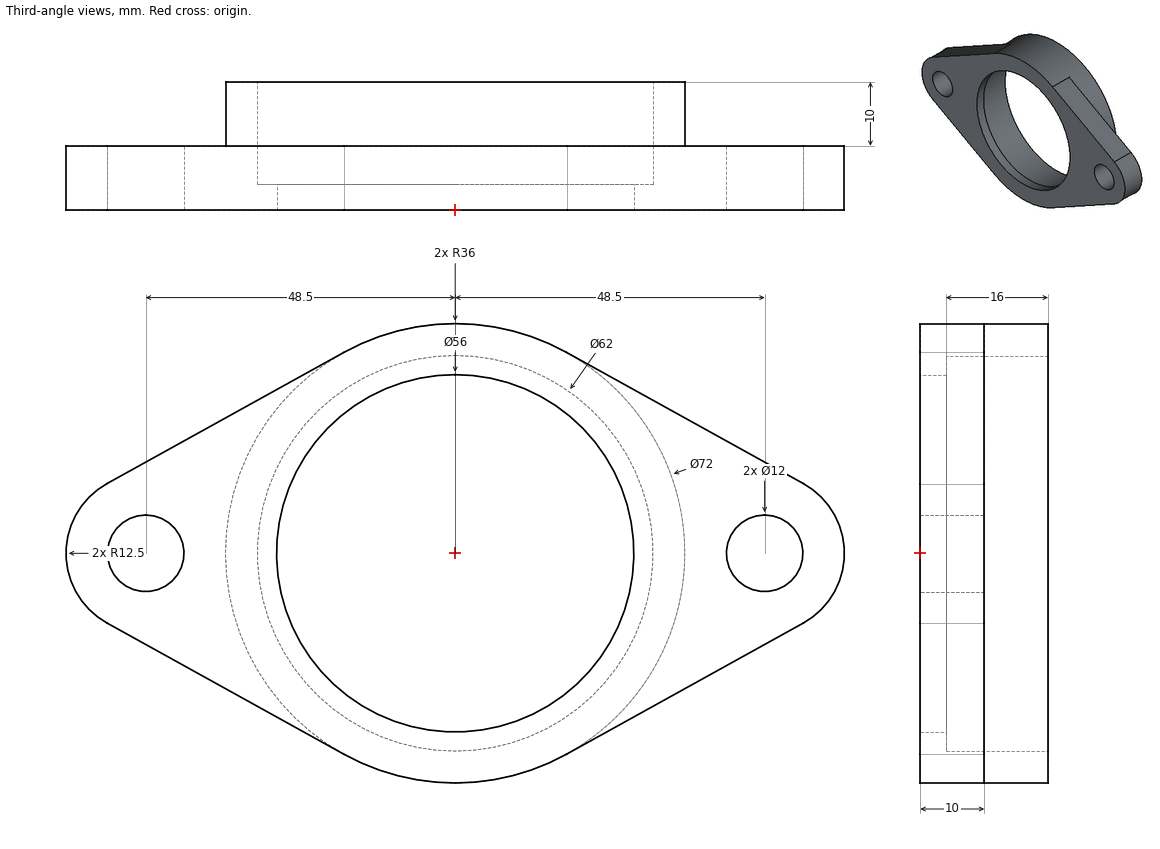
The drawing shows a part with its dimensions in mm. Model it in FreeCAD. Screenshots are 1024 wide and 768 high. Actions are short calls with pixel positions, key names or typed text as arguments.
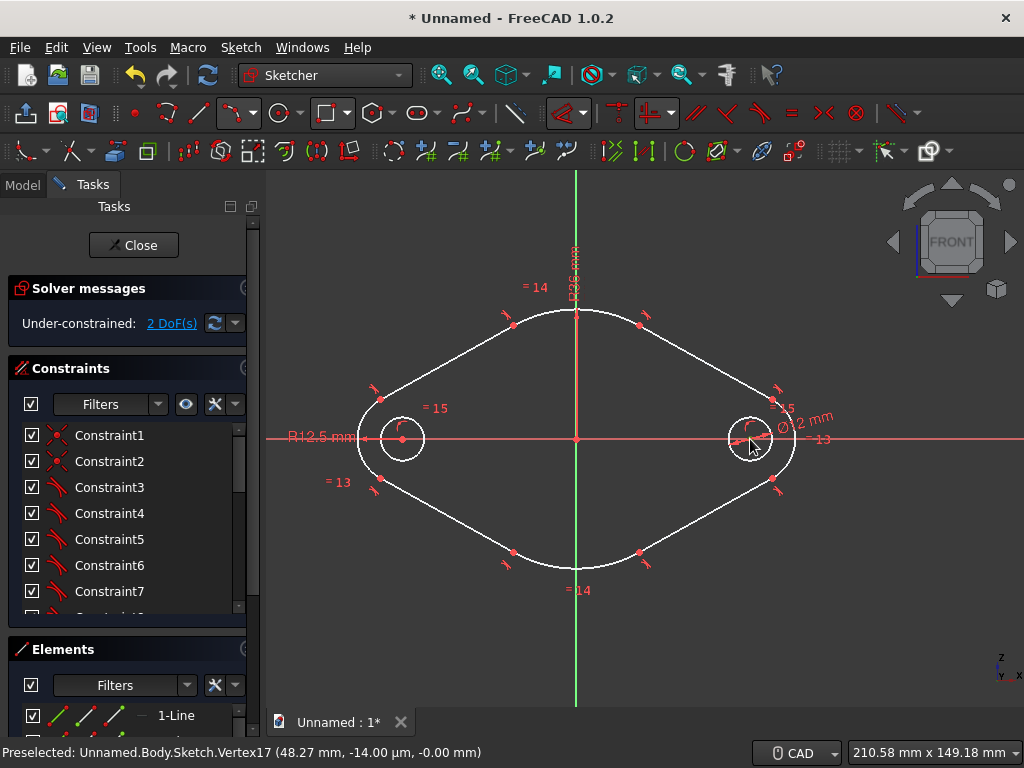
click(586, 114)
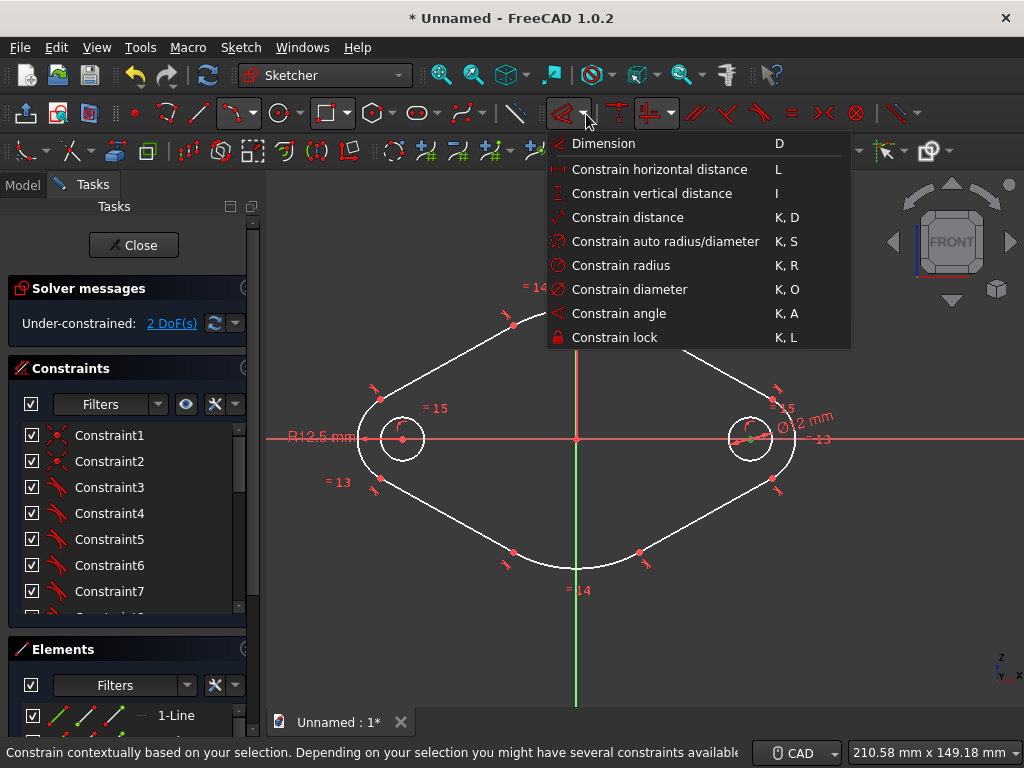
click(699, 169)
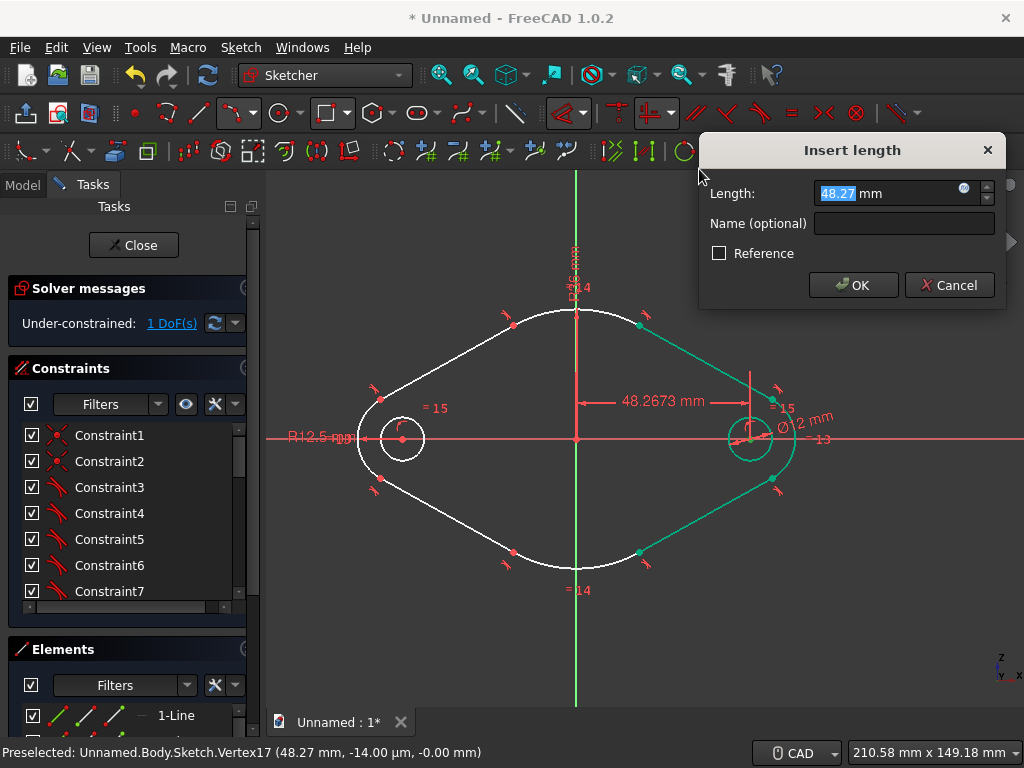
text(48.5)
key(Return)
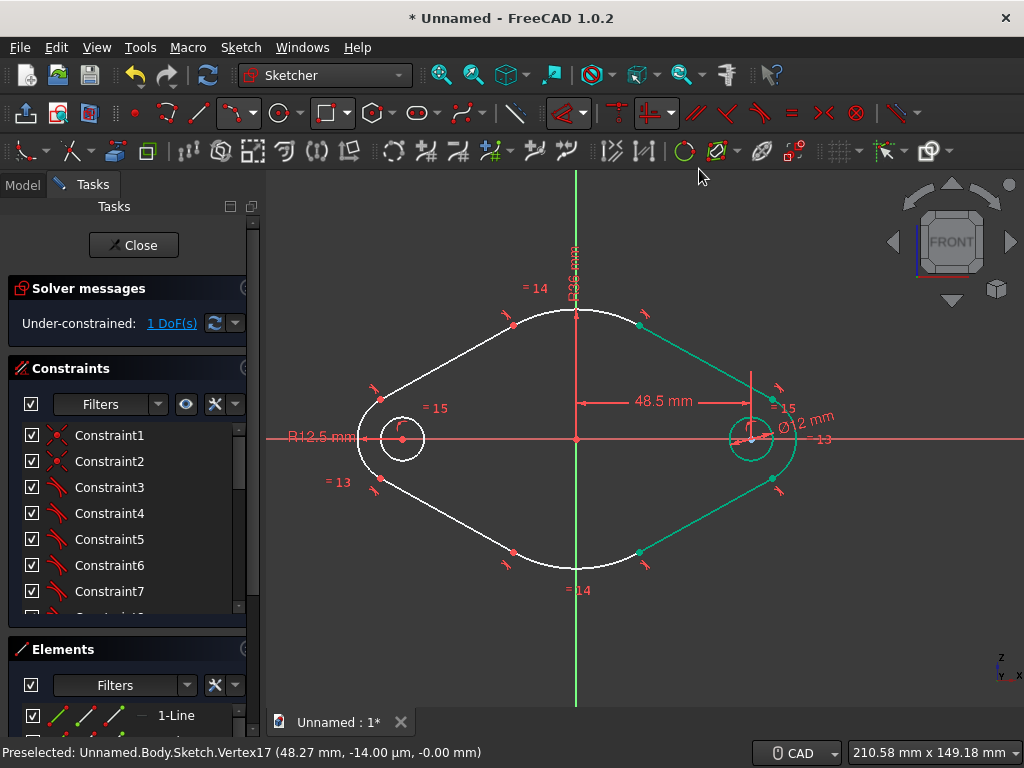
click(403, 439)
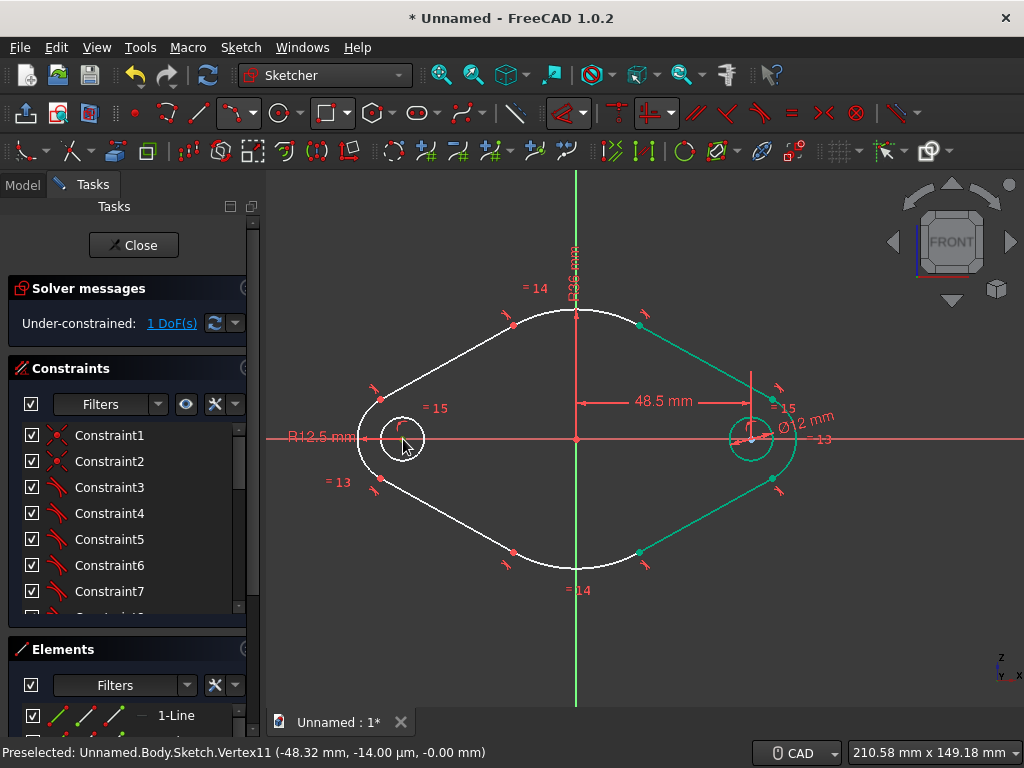
key(l)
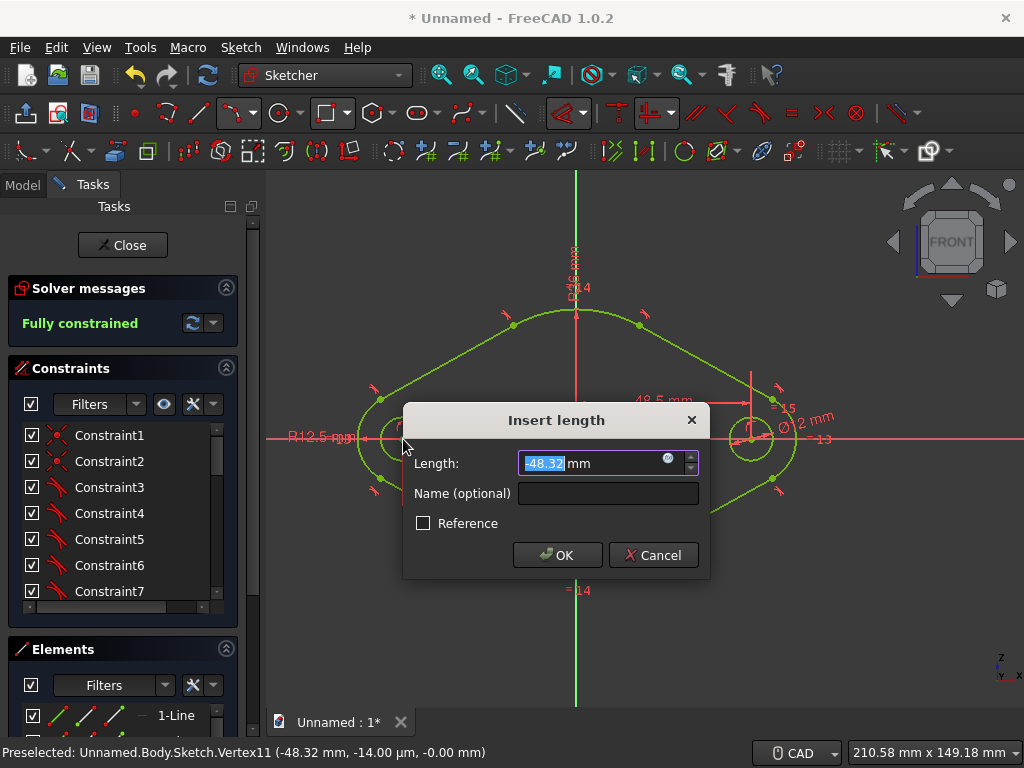
text(-48.5)
key(Return)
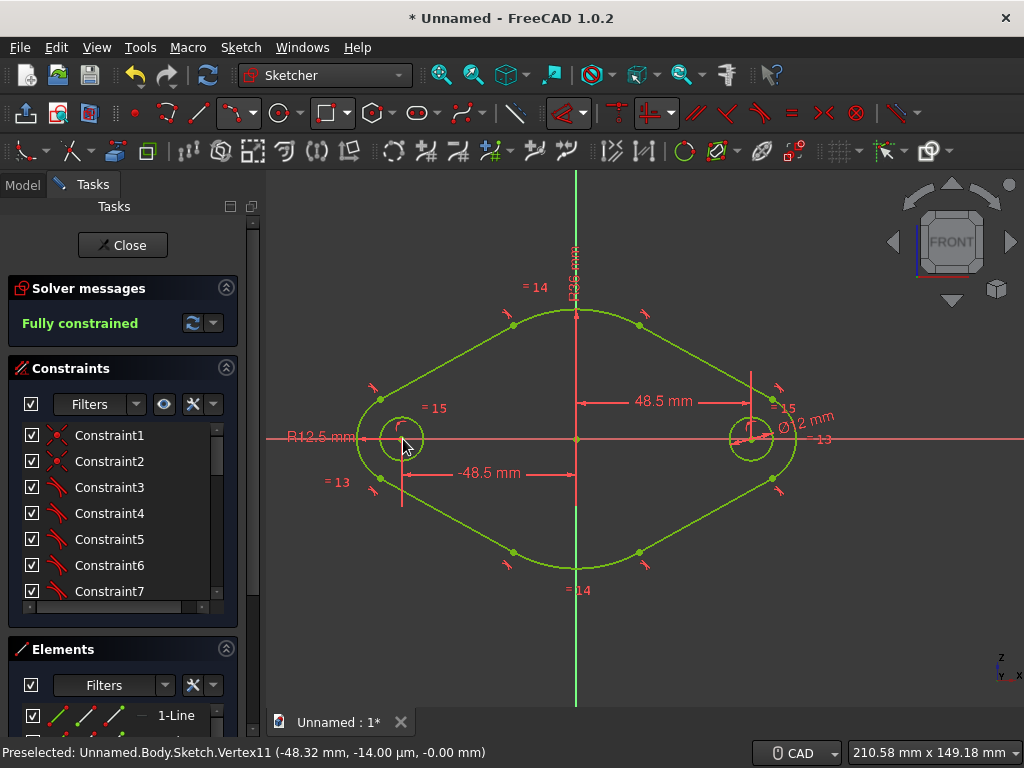
click(123, 245)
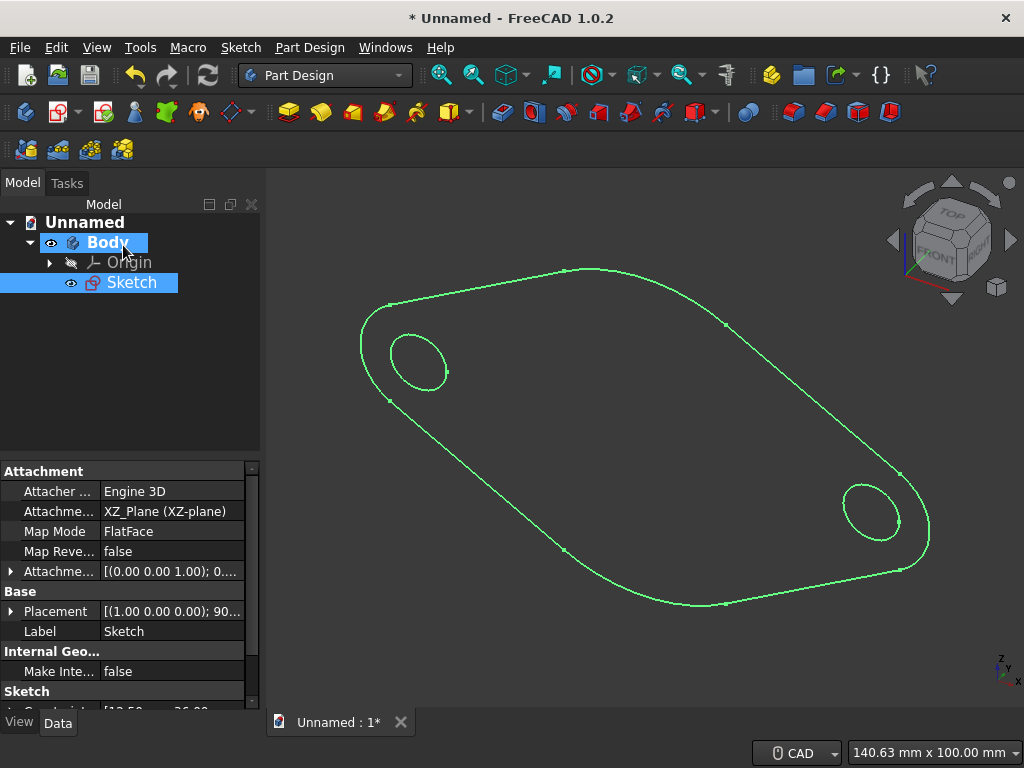
click(290, 112)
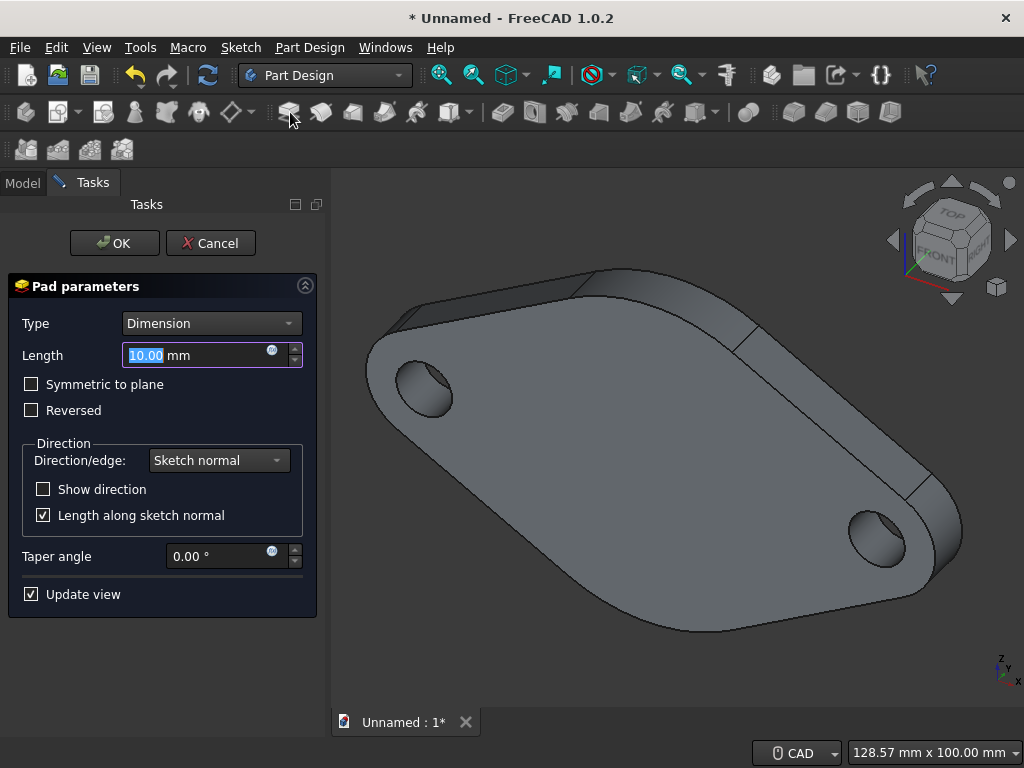
text(10)
key(Tab)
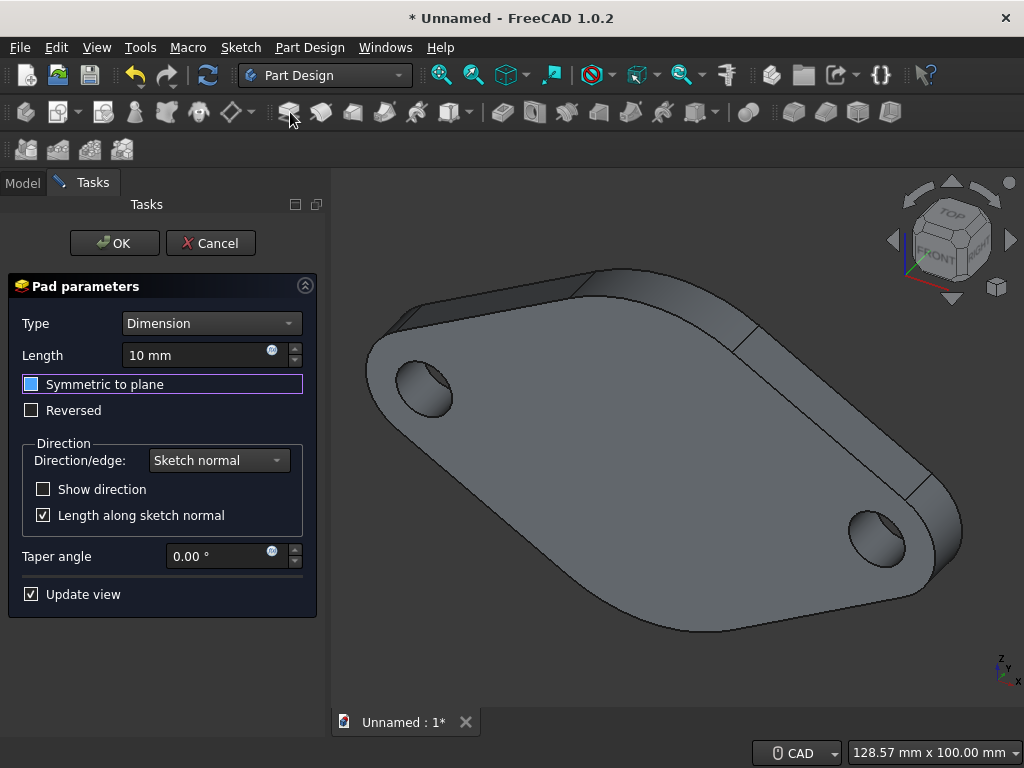
click(30, 410)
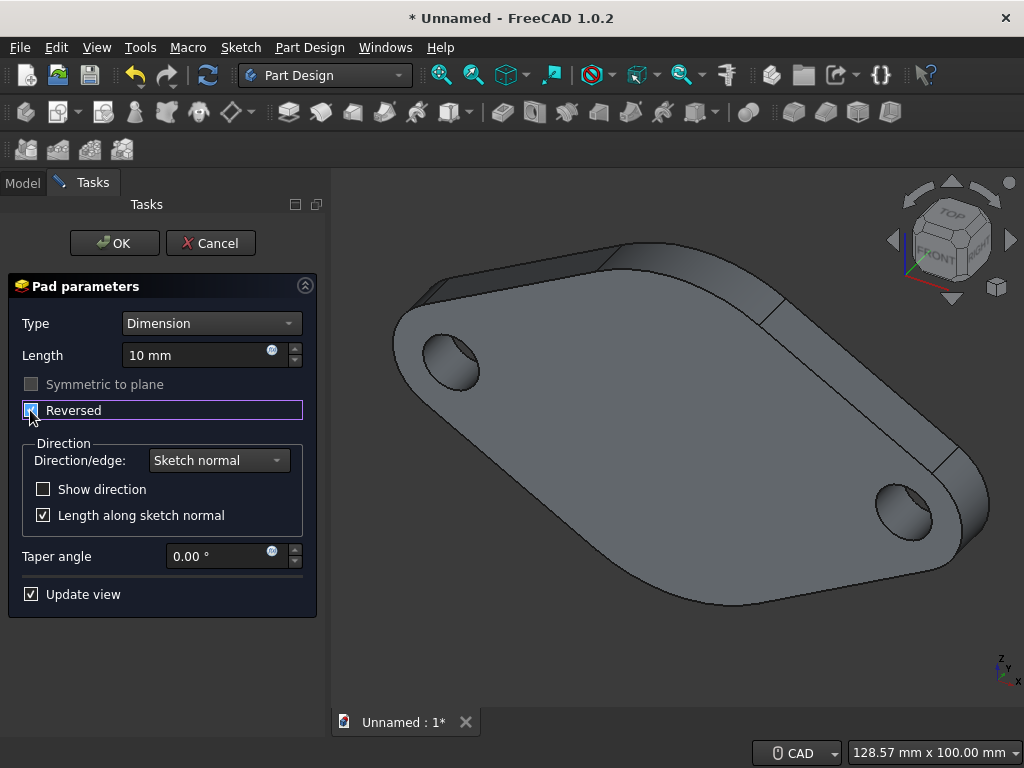
click(115, 243)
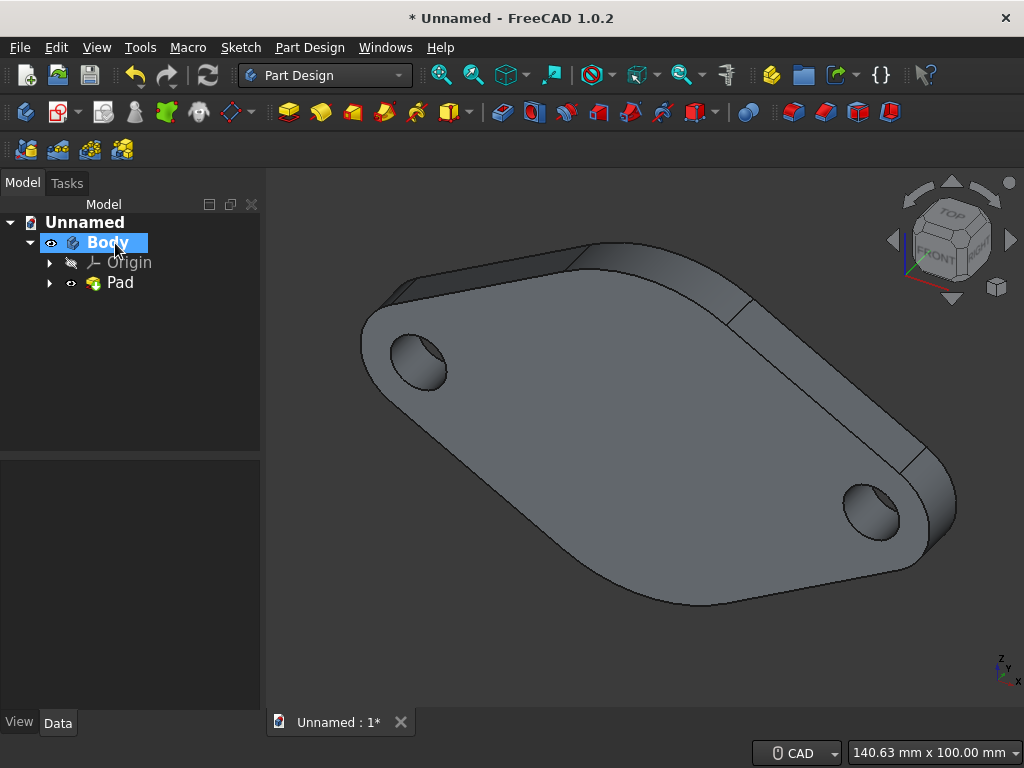
click(442, 76)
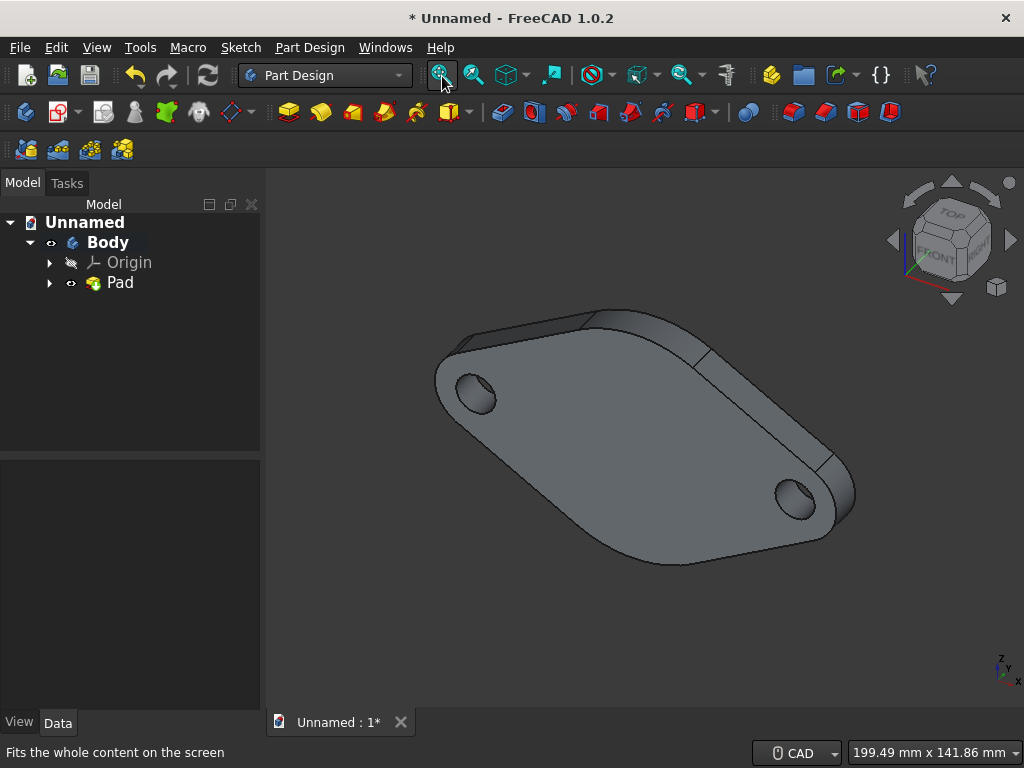
key(4)